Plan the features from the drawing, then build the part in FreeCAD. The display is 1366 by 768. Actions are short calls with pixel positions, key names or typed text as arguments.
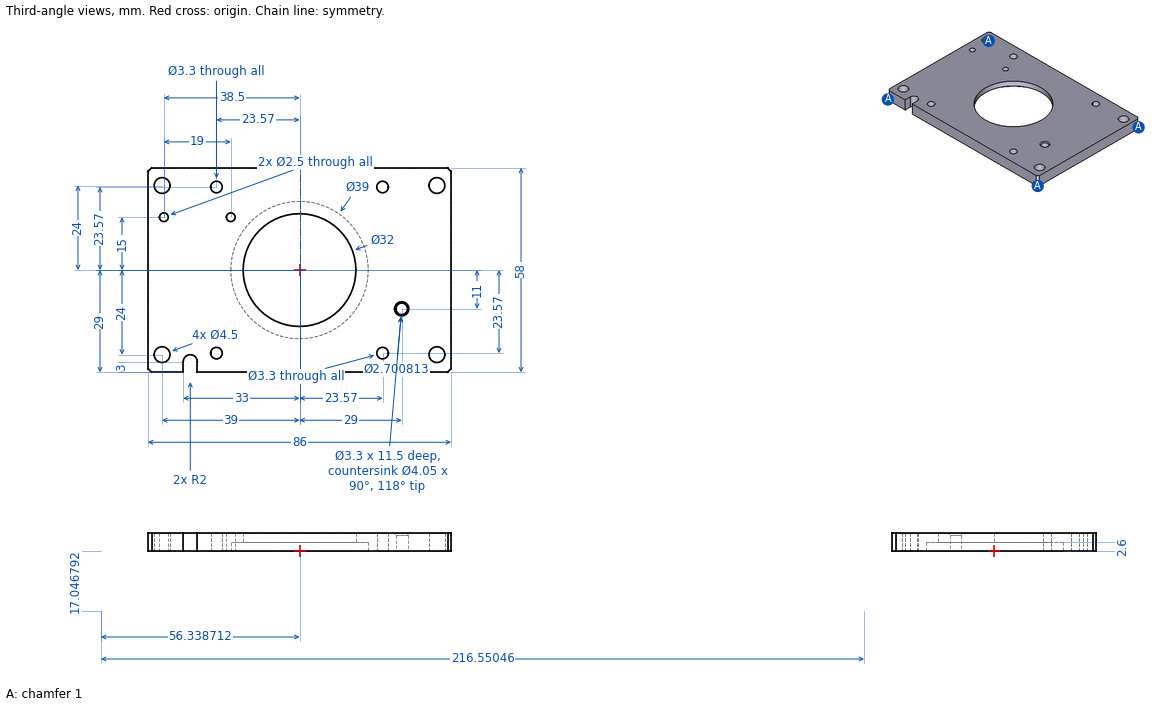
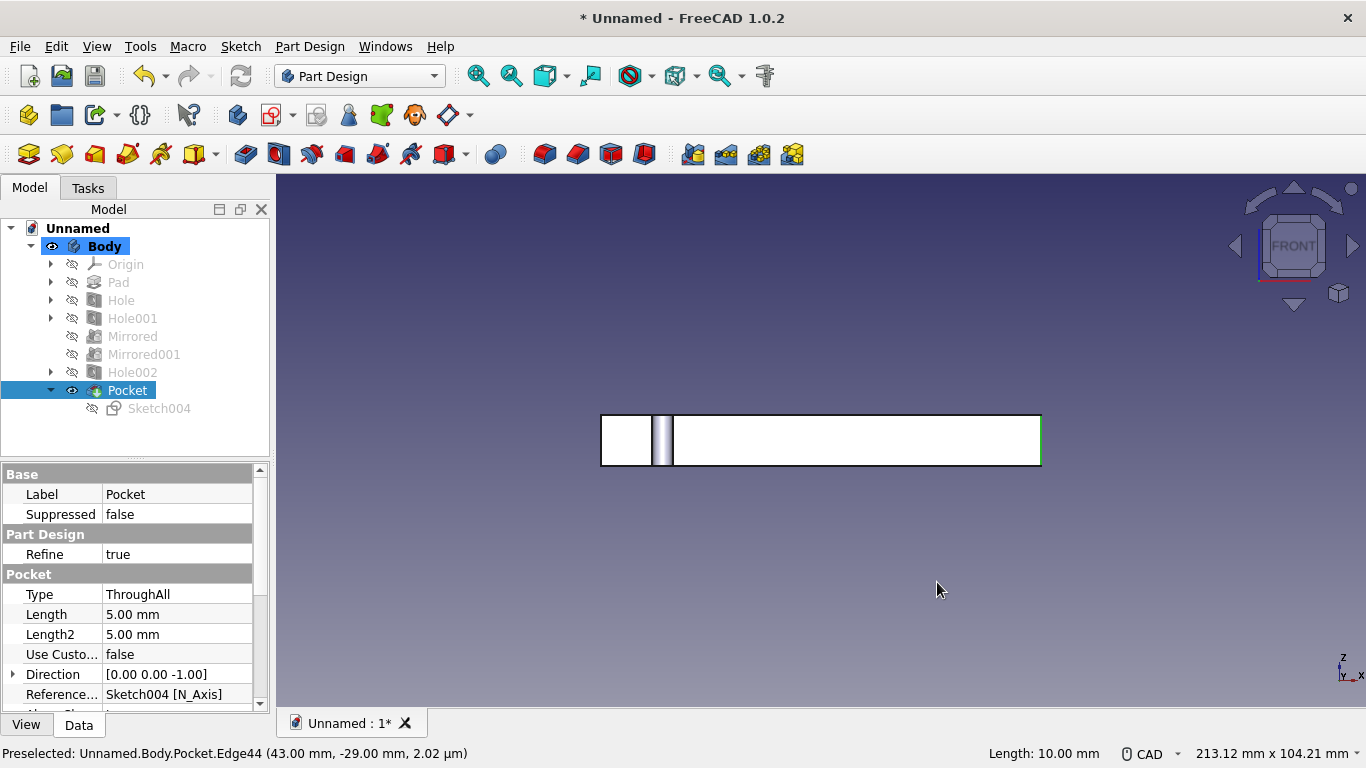
click(601, 440, ctrl)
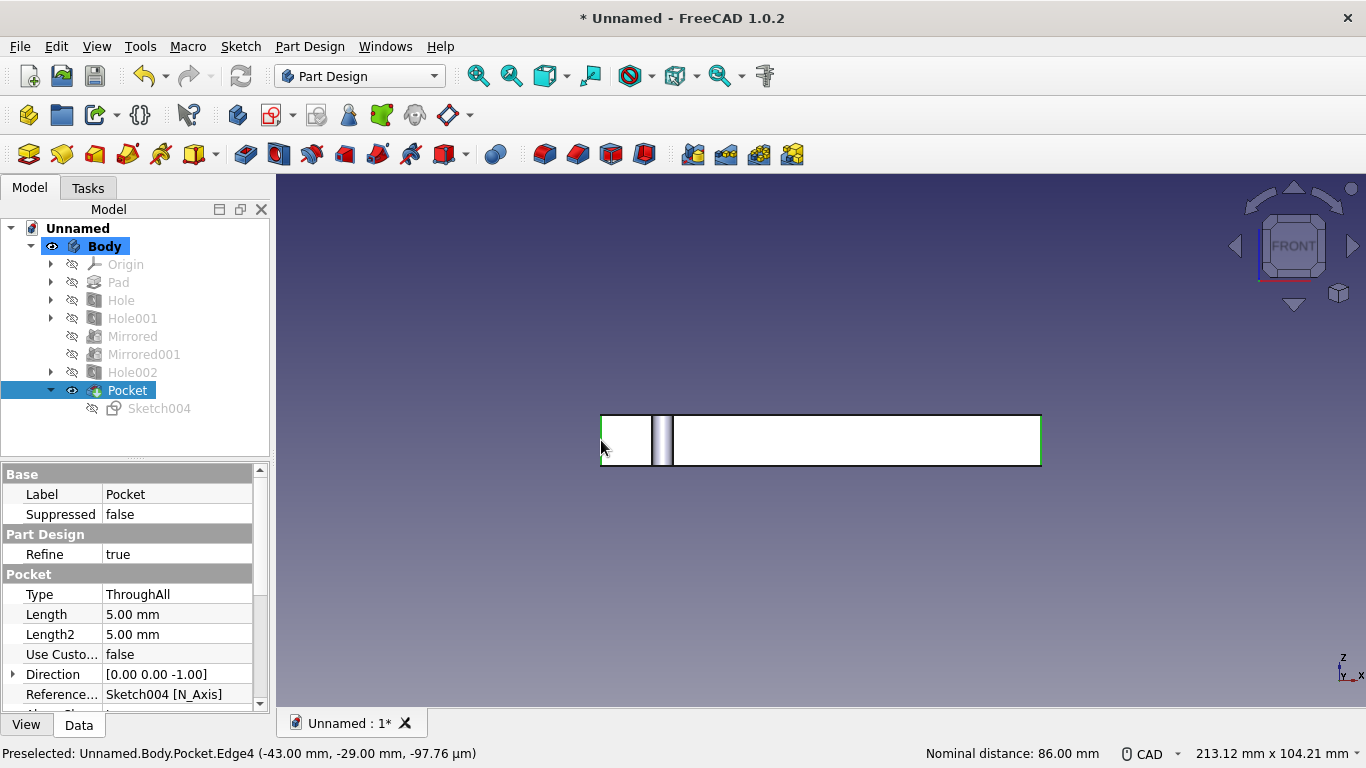
key(3)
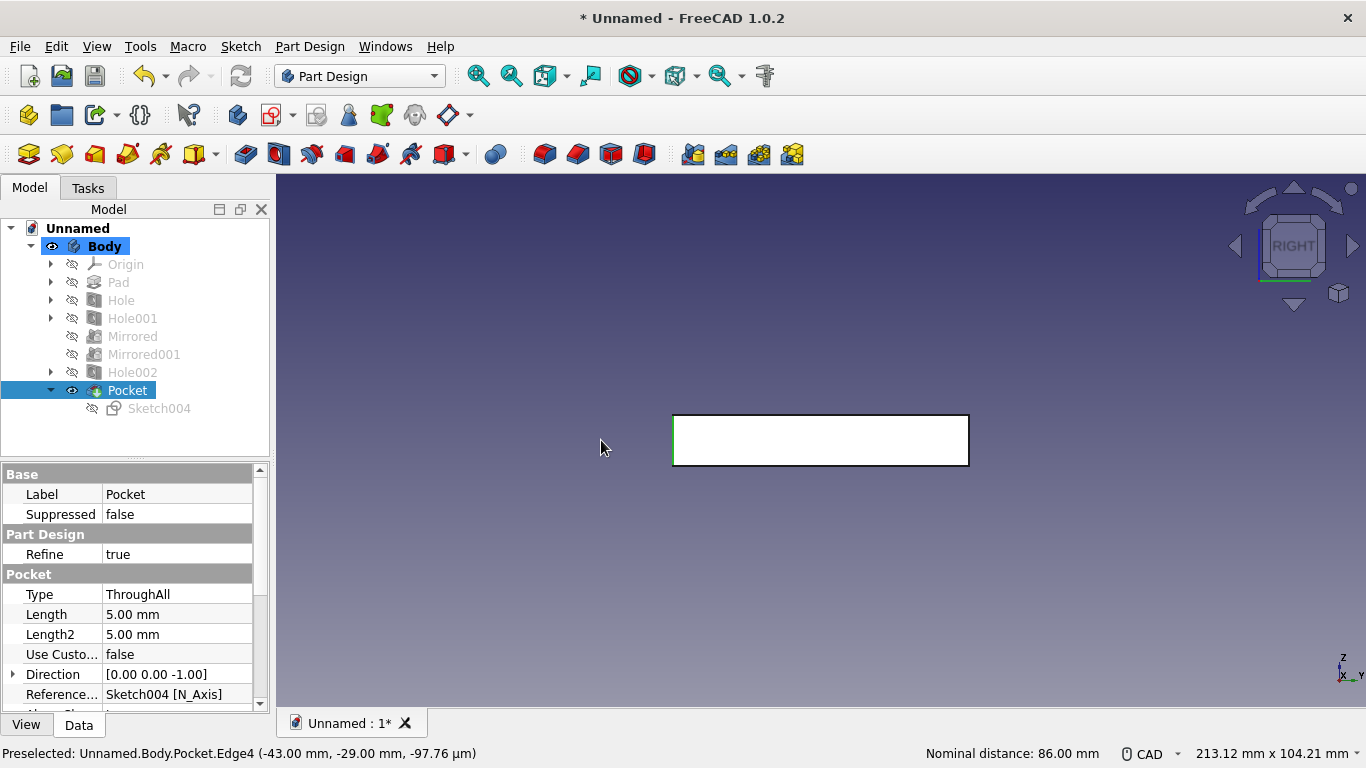
click(479, 76)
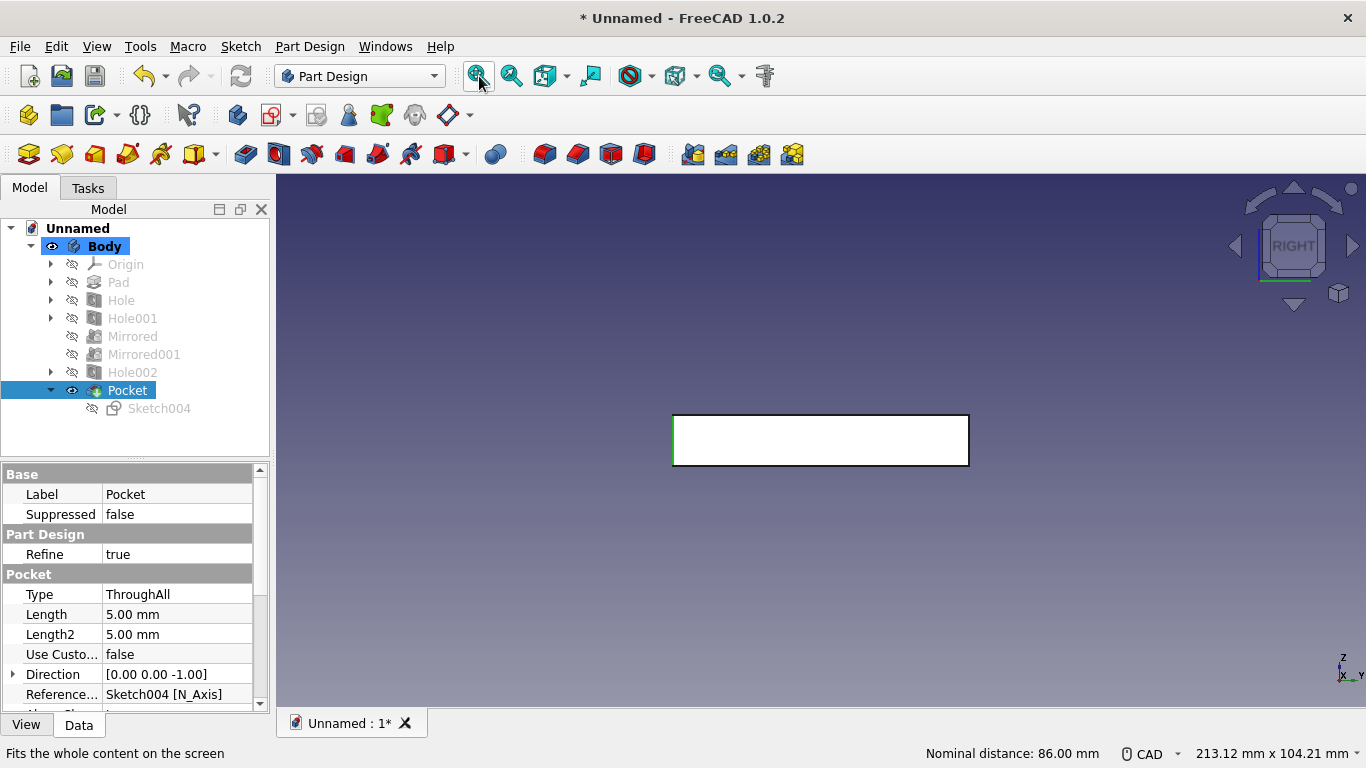
click(969, 439, ctrl)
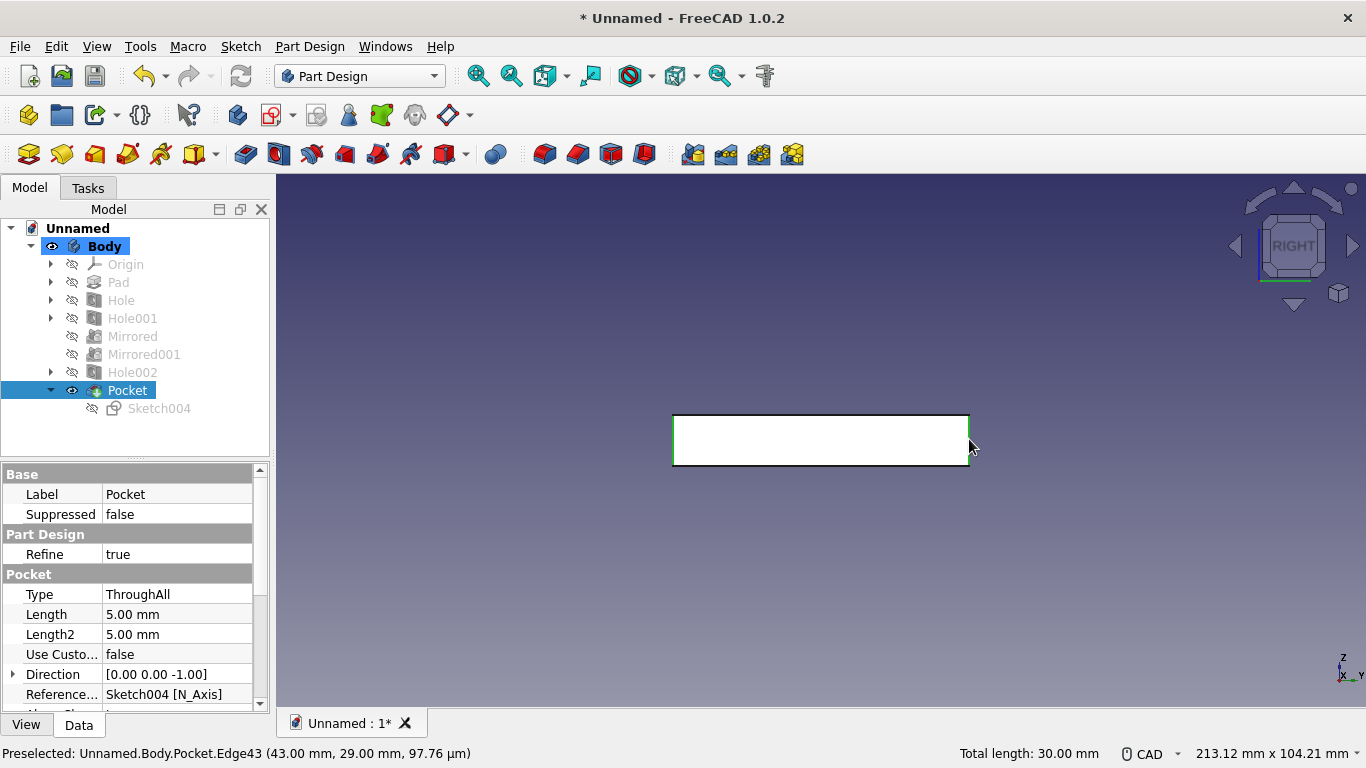
key(5)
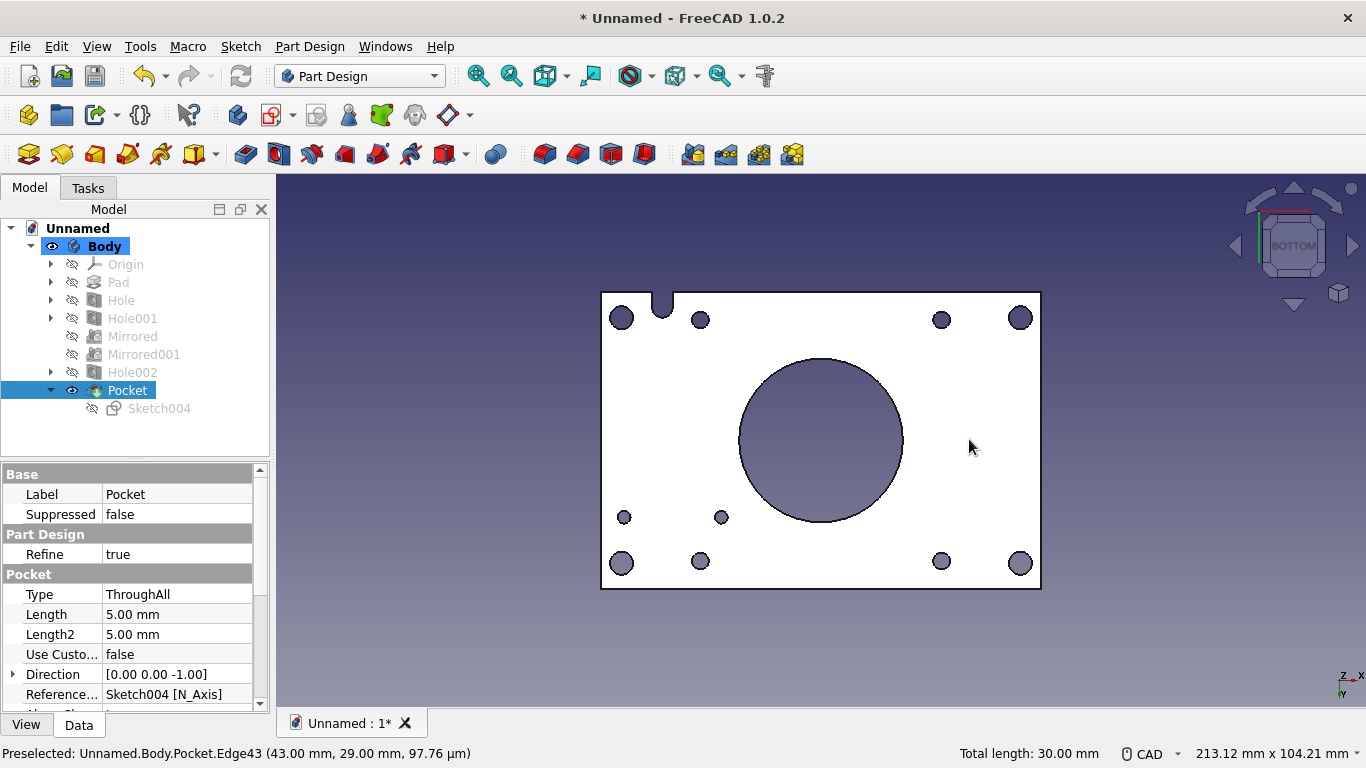
key(4)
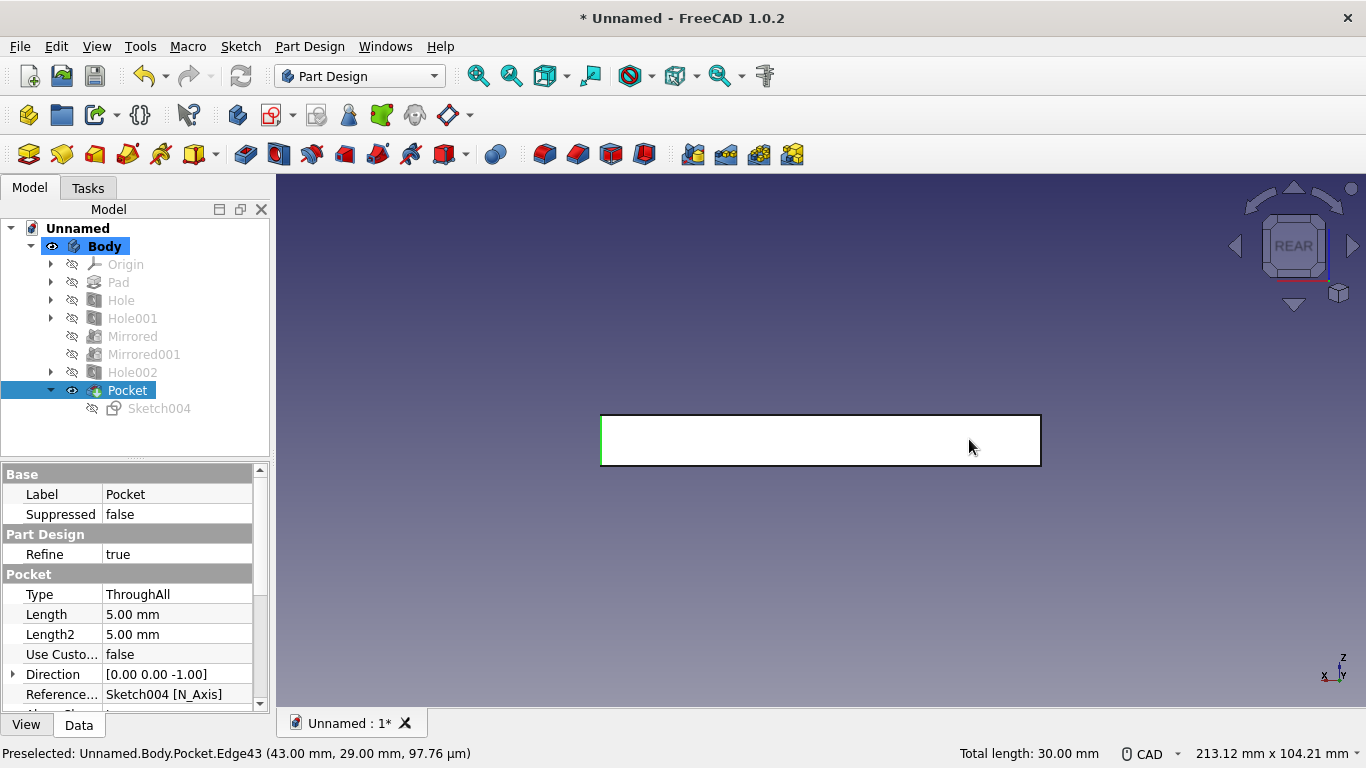
click(479, 76)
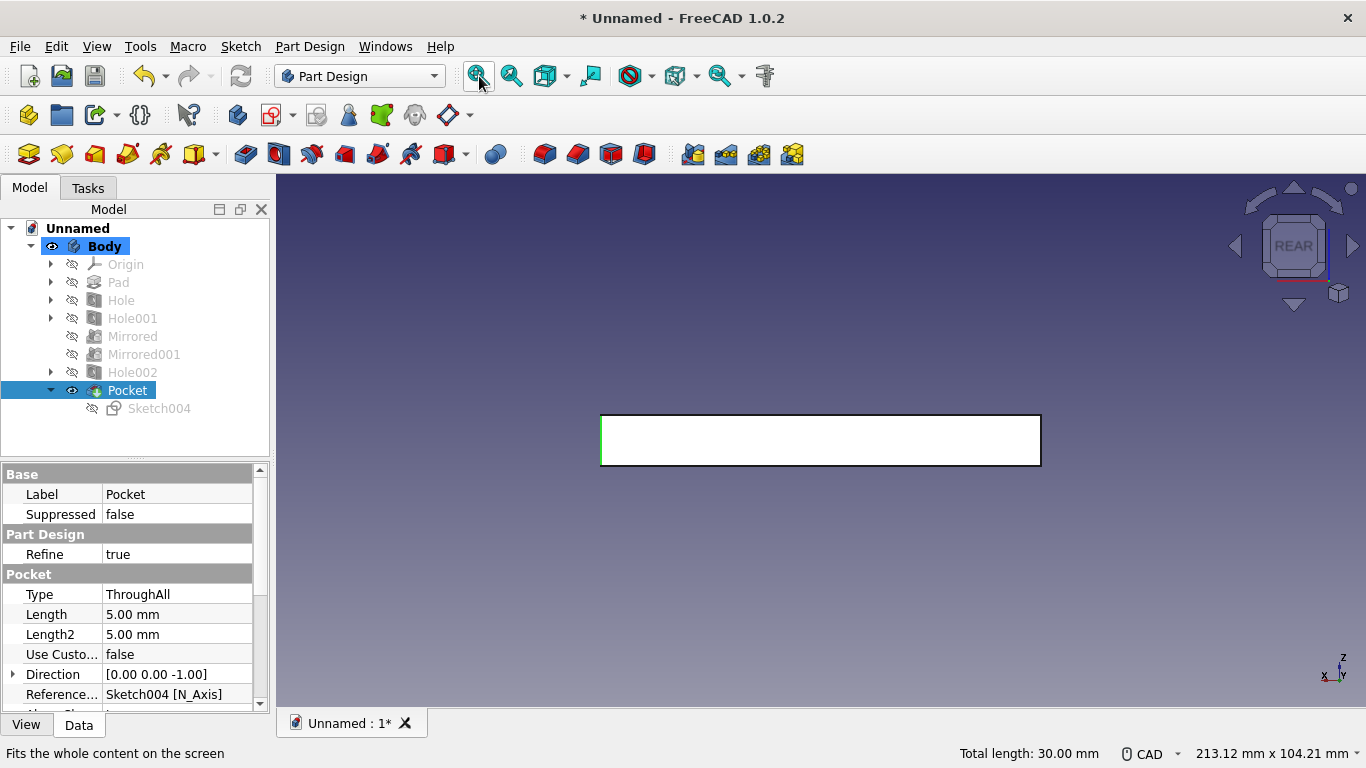
click(1041, 440, ctrl)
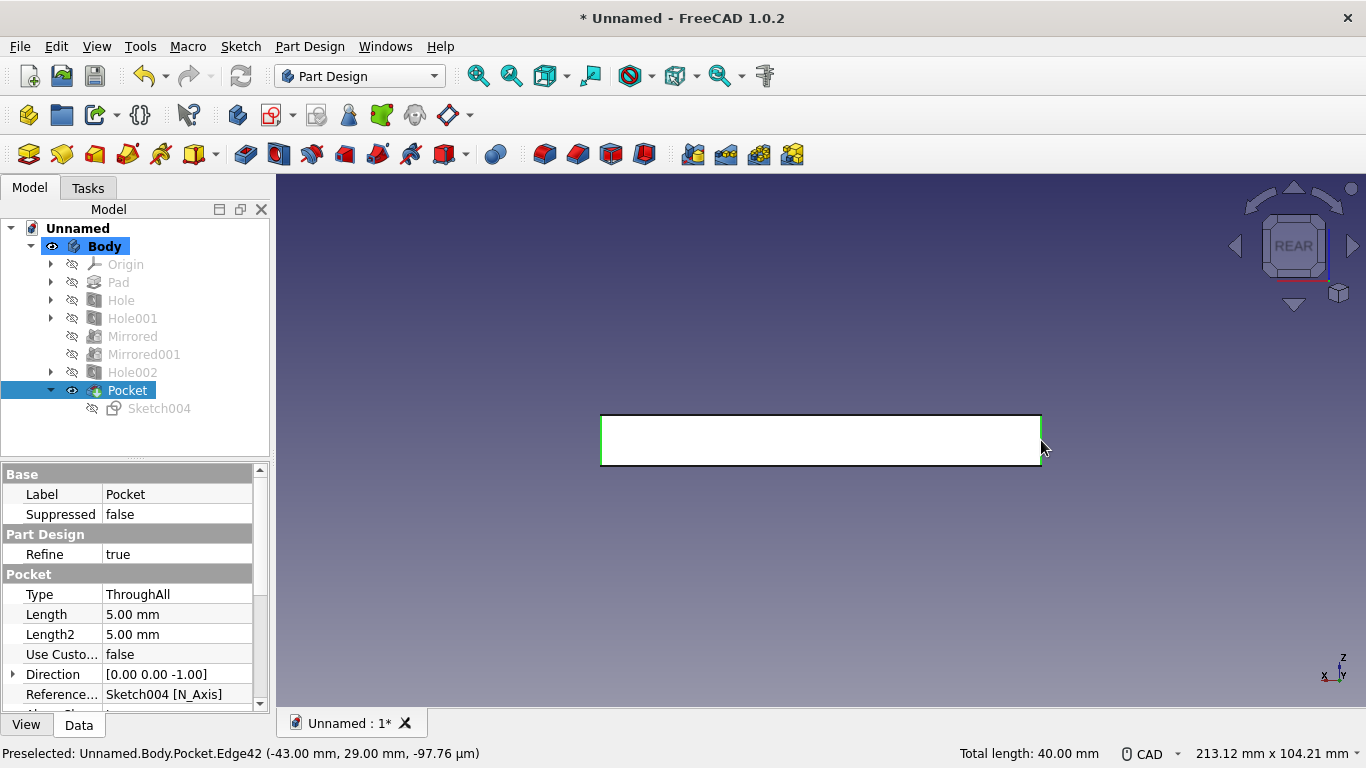
click(578, 154)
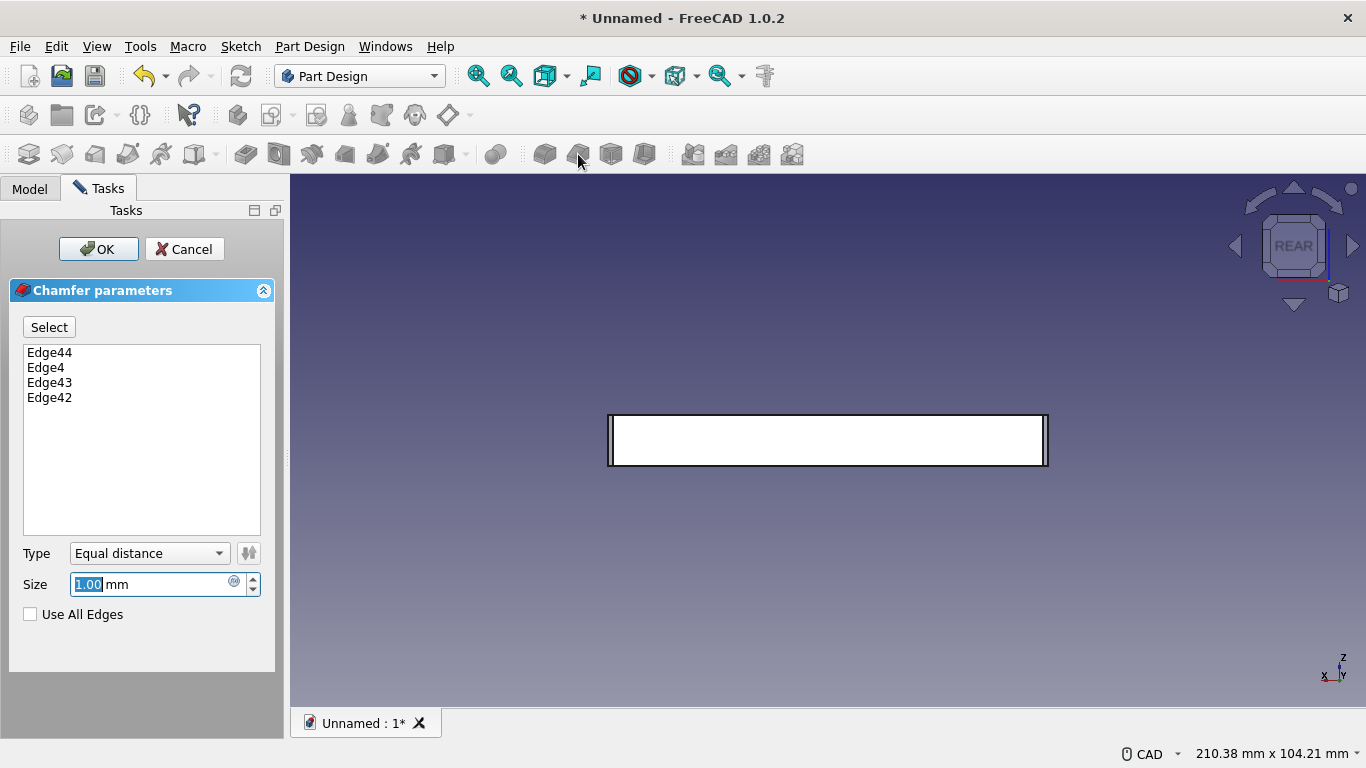
text(1)
key(Tab)